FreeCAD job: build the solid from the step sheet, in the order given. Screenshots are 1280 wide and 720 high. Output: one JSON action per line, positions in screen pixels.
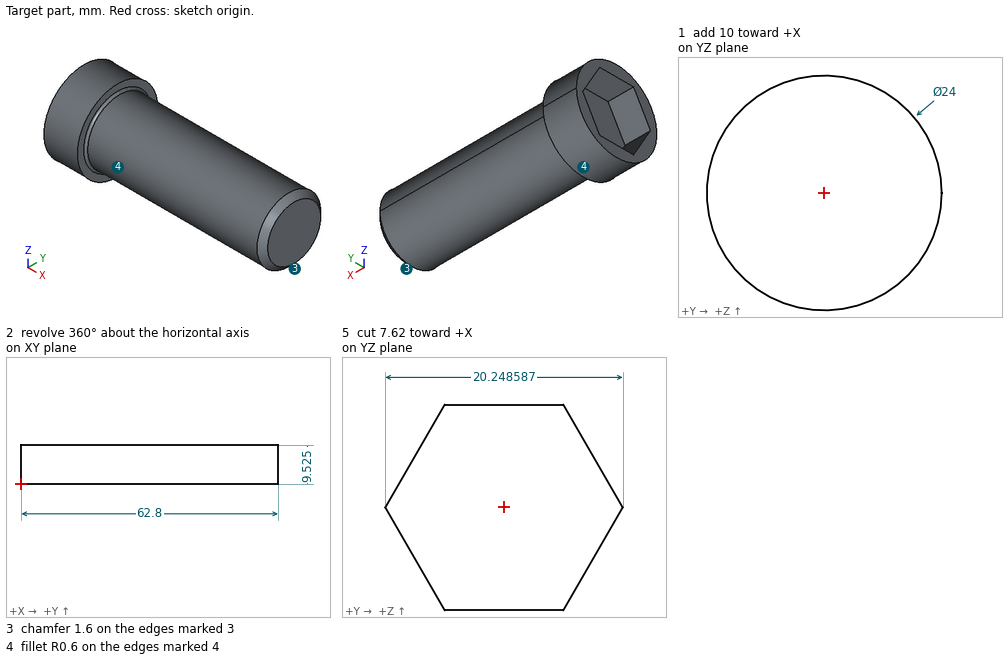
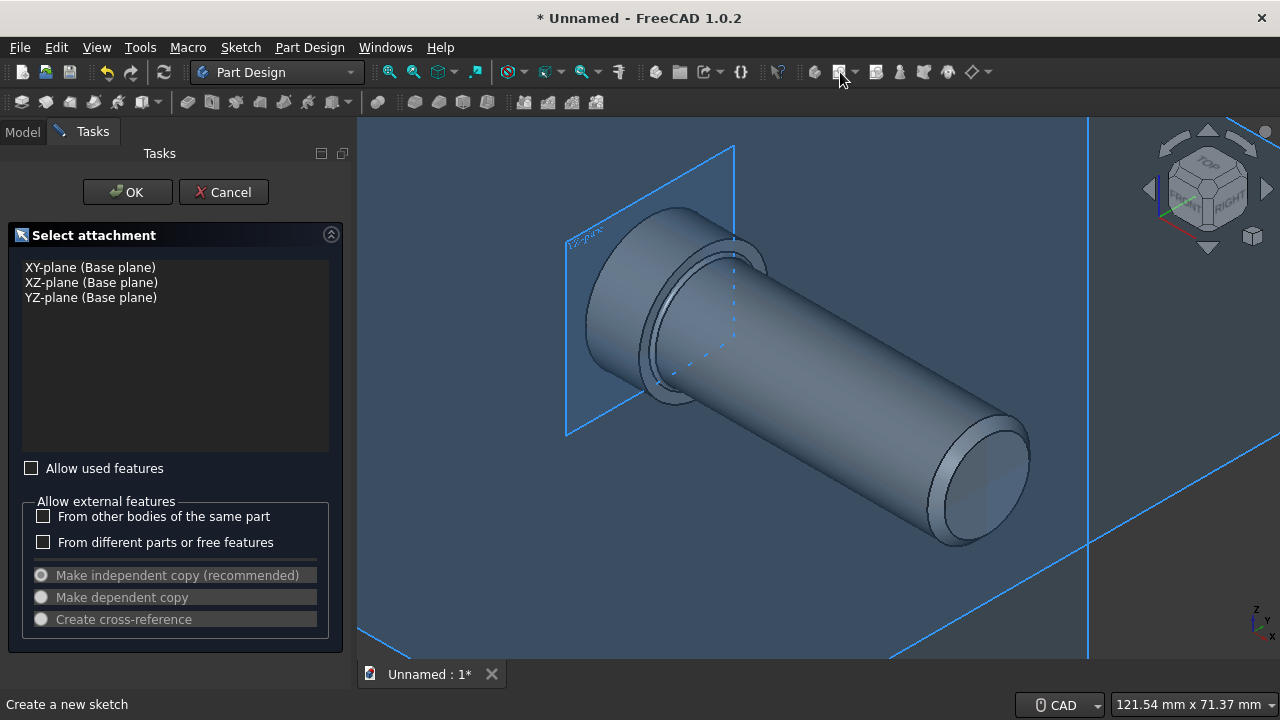
{"action": "left_click", "coordinate": [82, 298]}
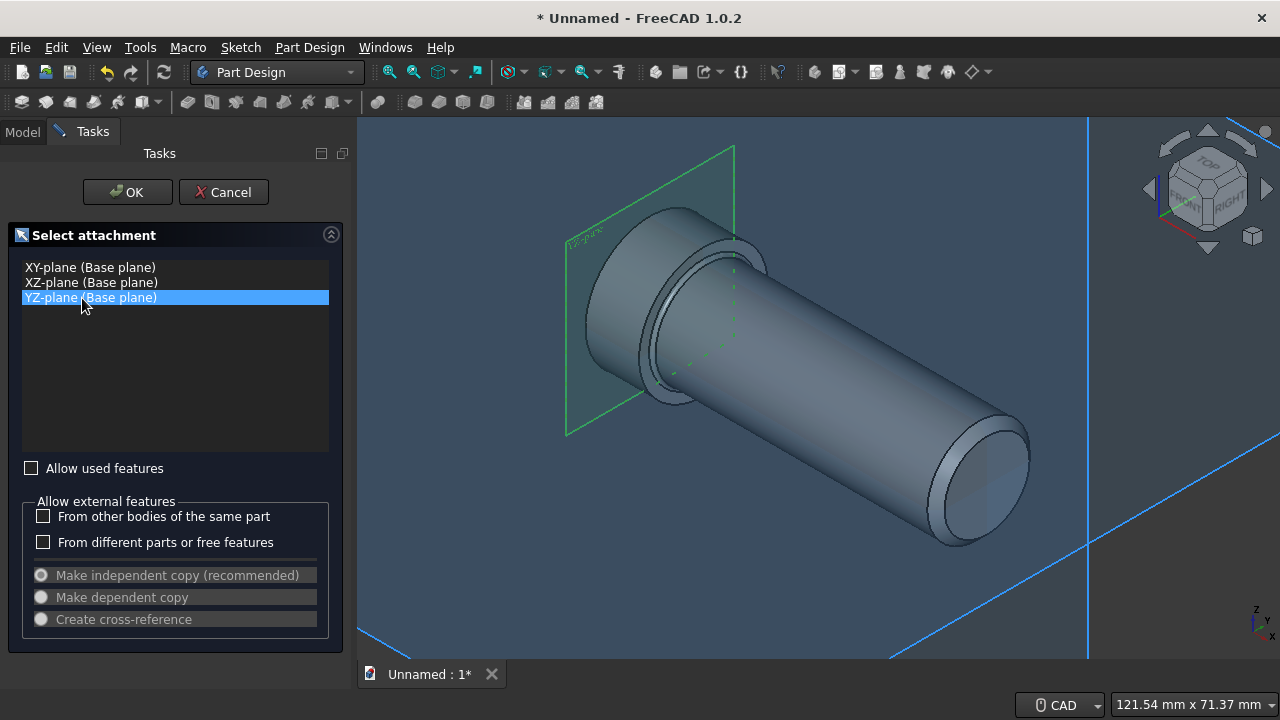
{"action": "left_click", "coordinate": [128, 192]}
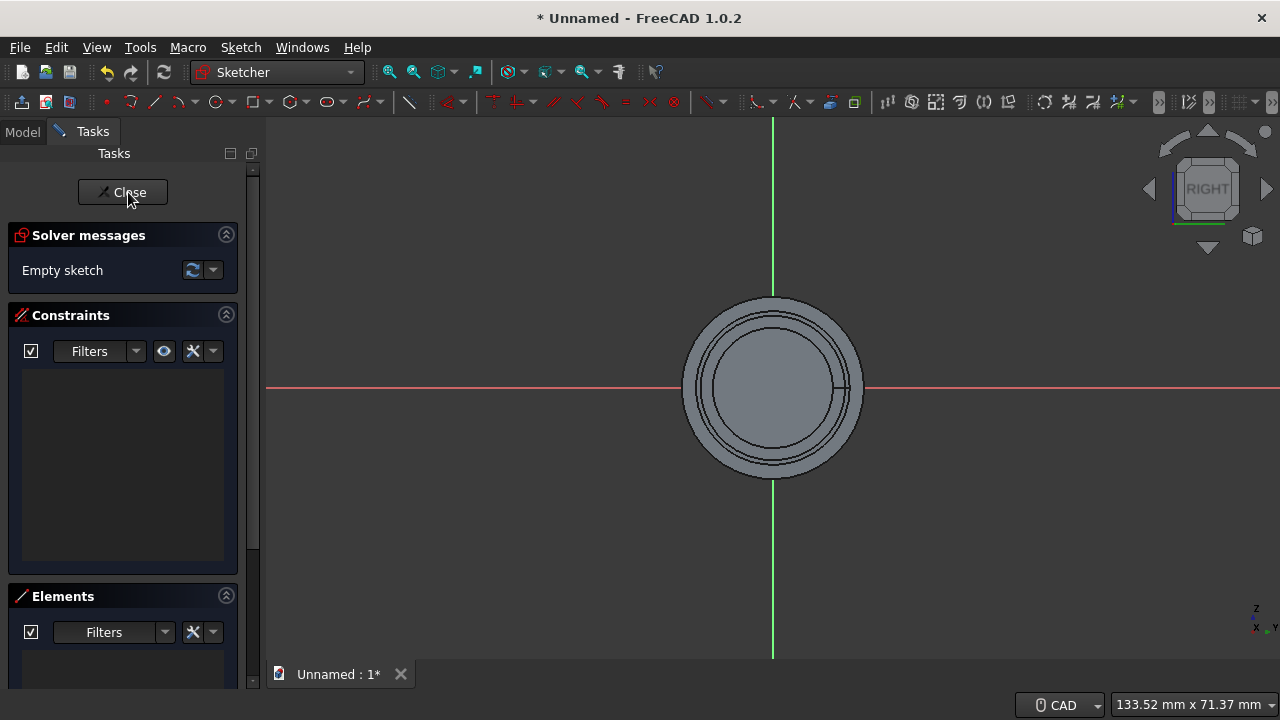
{"action": "left_click", "coordinate": [70, 102]}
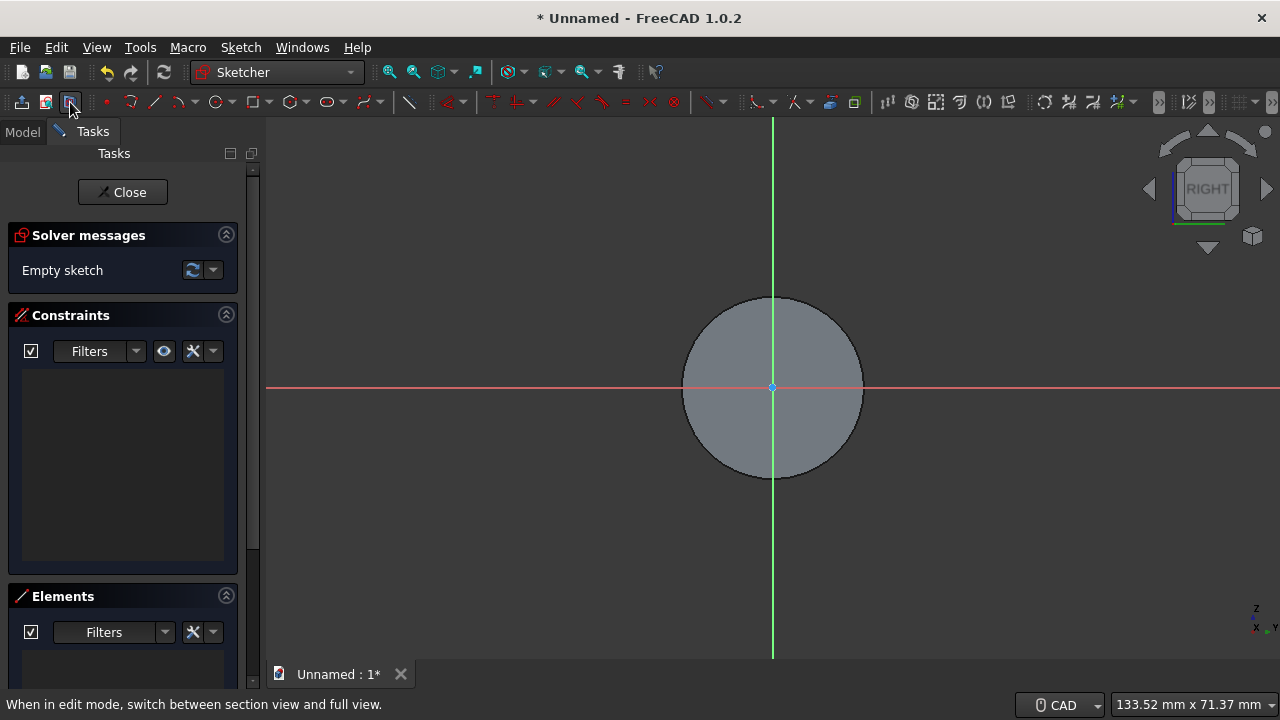
{"action": "scroll", "coordinate": [813, 388], "scroll_direction": "up", "scroll_amount": 5}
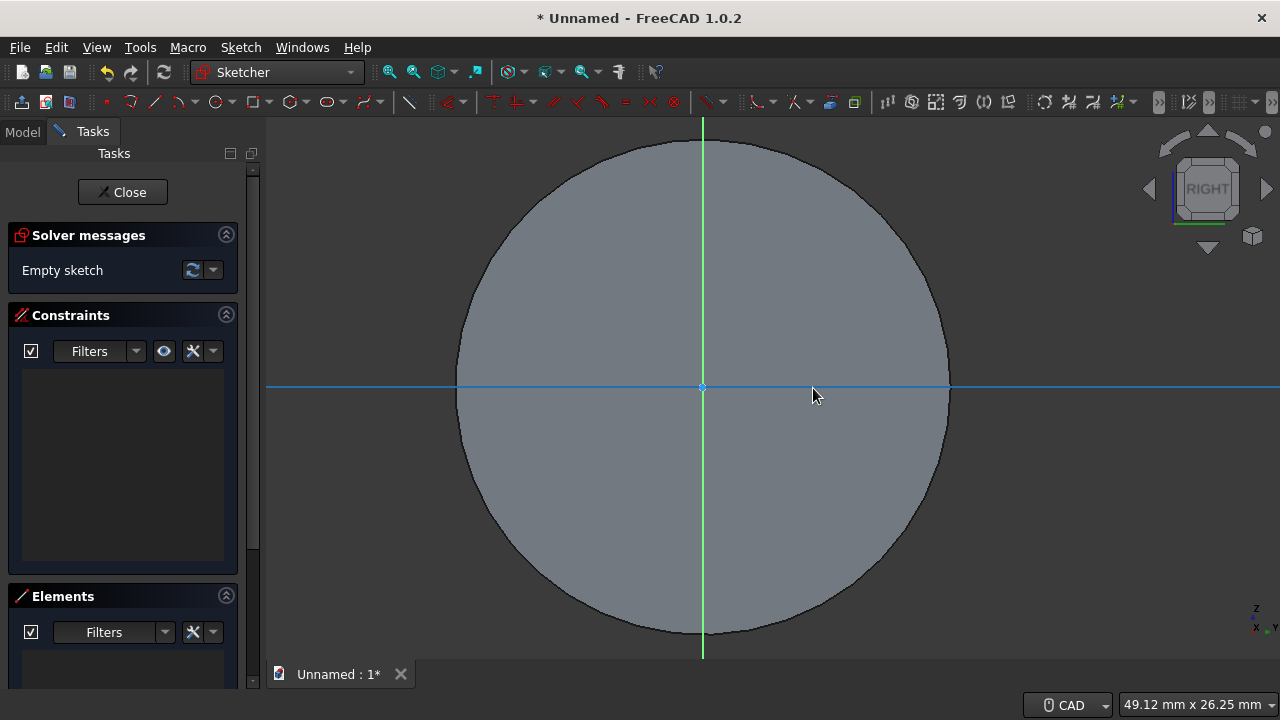
{"action": "left_click", "coordinate": [290, 102]}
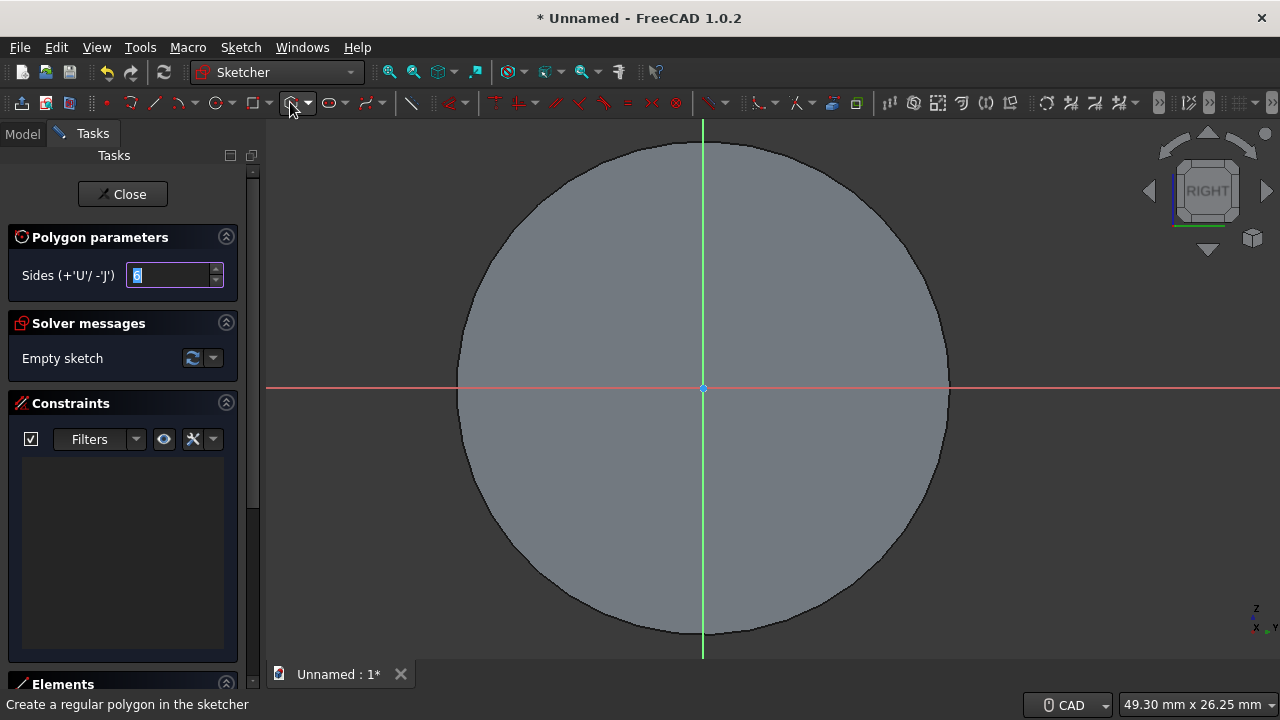
{"action": "left_click", "coordinate": [703, 388]}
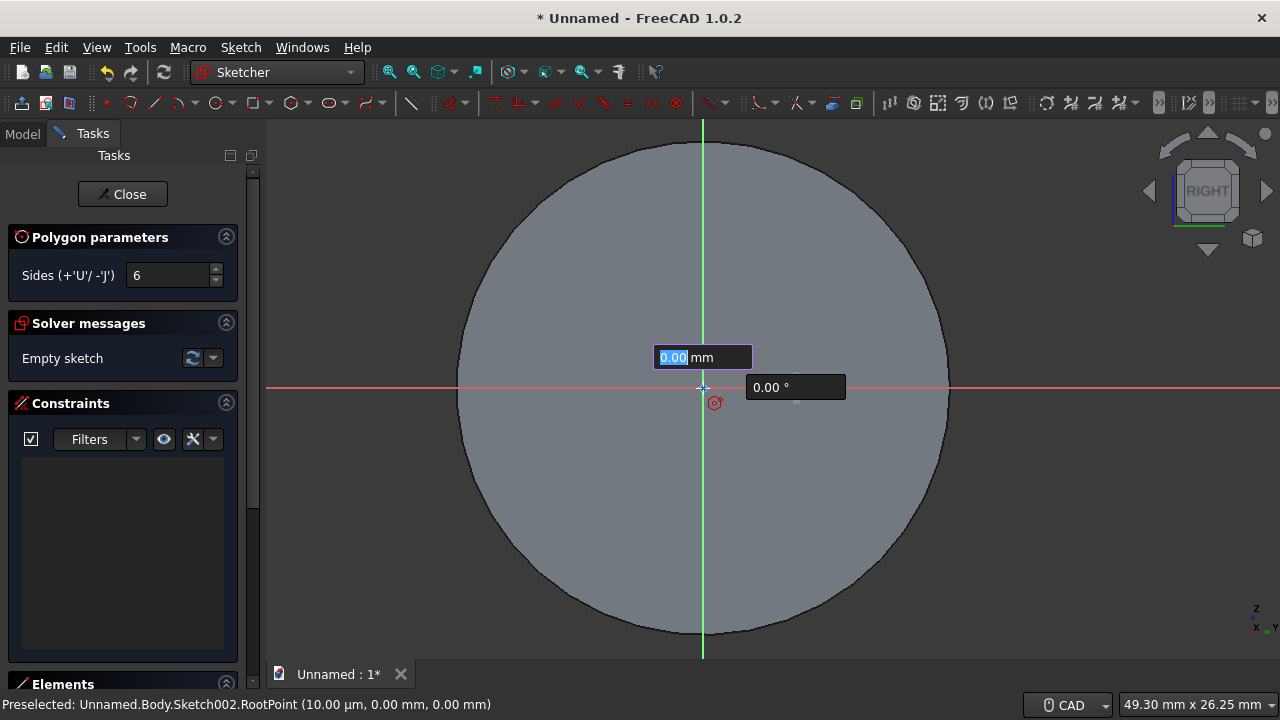
{"action": "left_click", "coordinate": [495, 388]}
{"action": "right_click", "coordinate": [495, 388]}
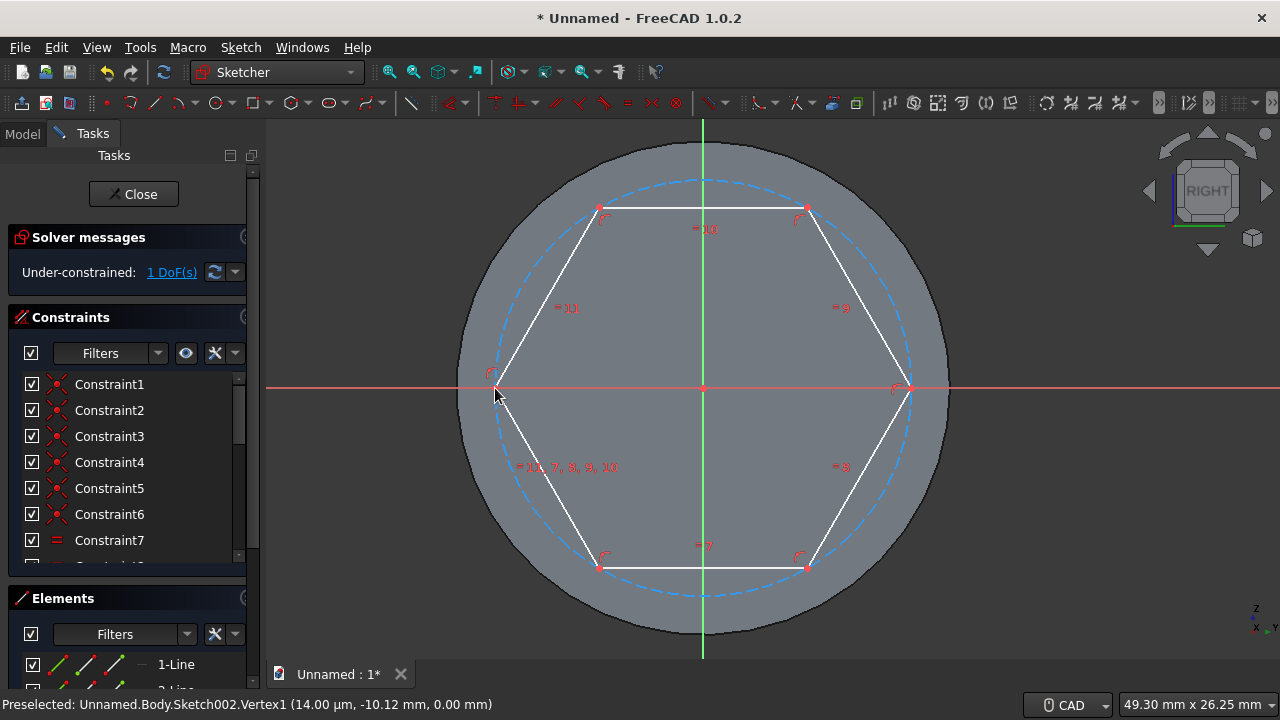
{"action": "left_click", "coordinate": [495, 388]}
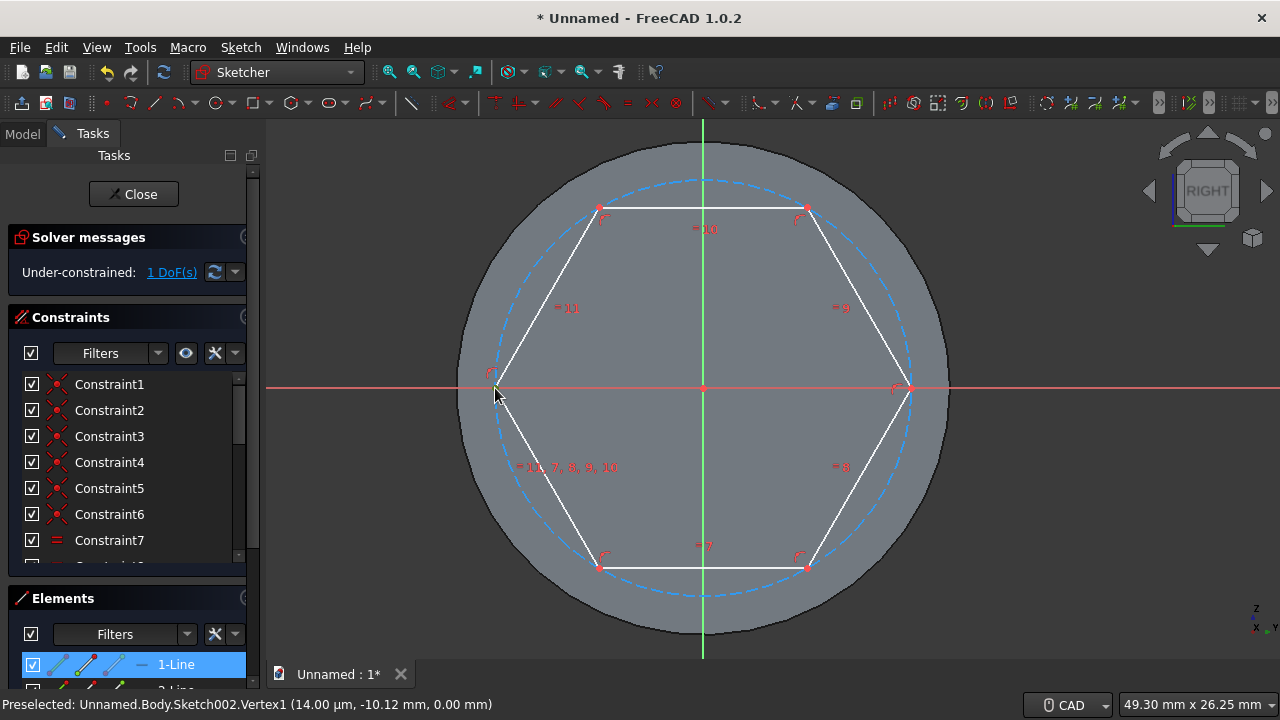
{"action": "left_click", "coordinate": [911, 388]}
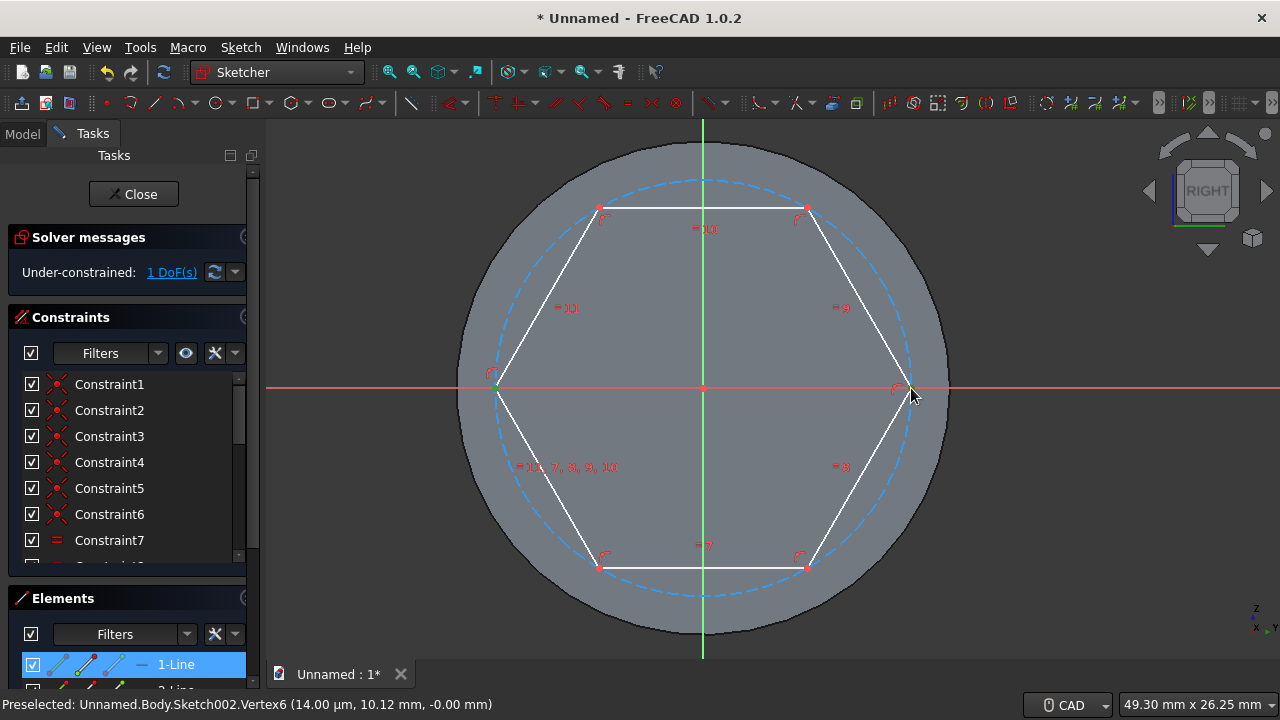
{"action": "left_click", "coordinate": [468, 104]}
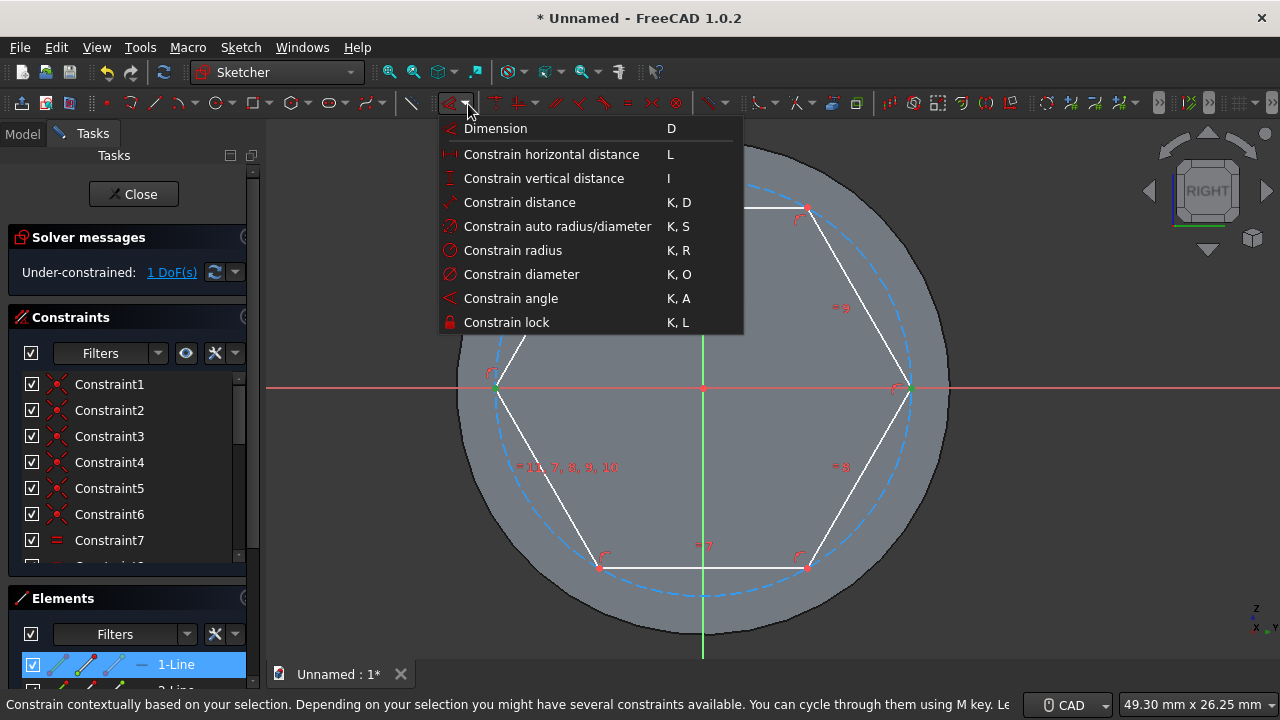
{"action": "left_click", "coordinate": [591, 154]}